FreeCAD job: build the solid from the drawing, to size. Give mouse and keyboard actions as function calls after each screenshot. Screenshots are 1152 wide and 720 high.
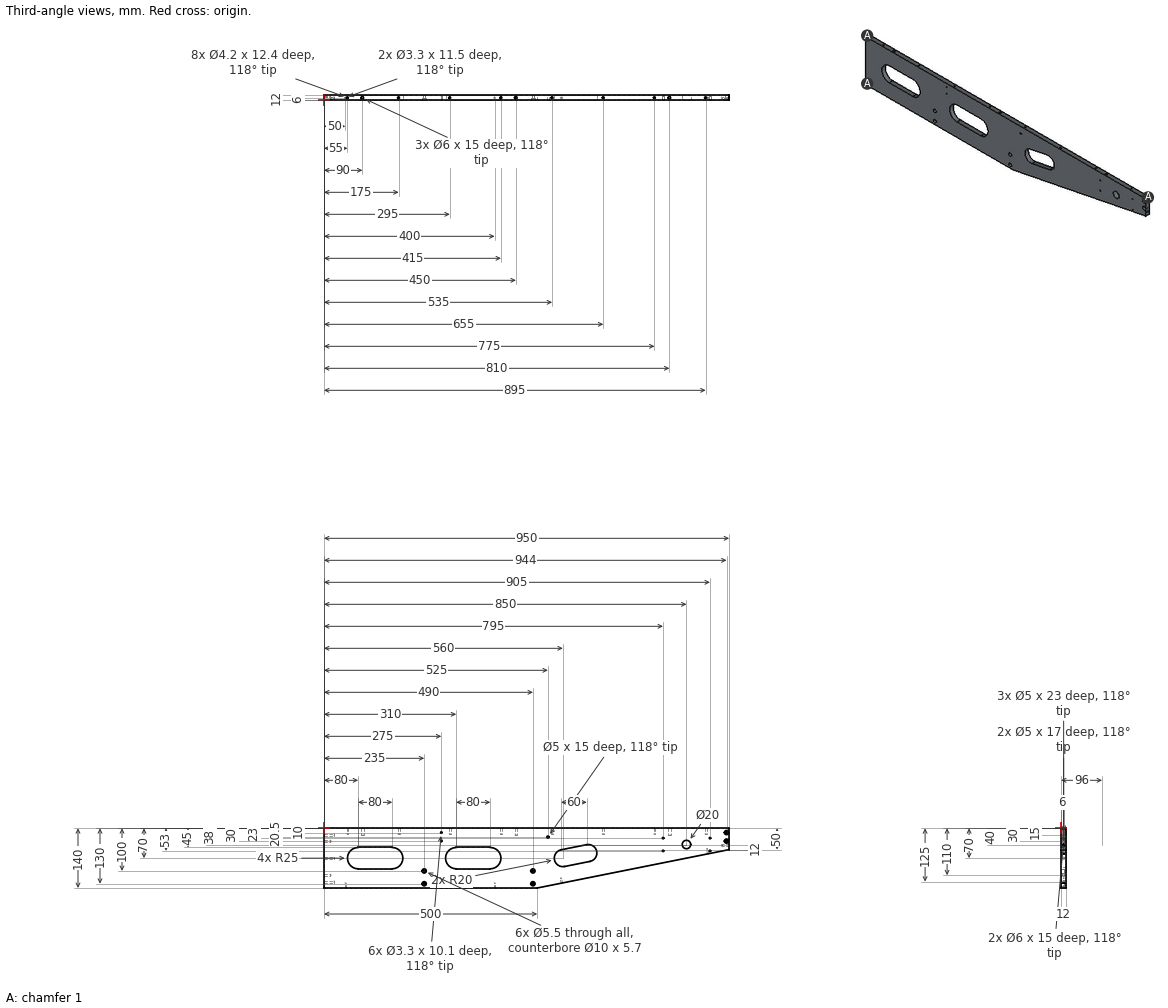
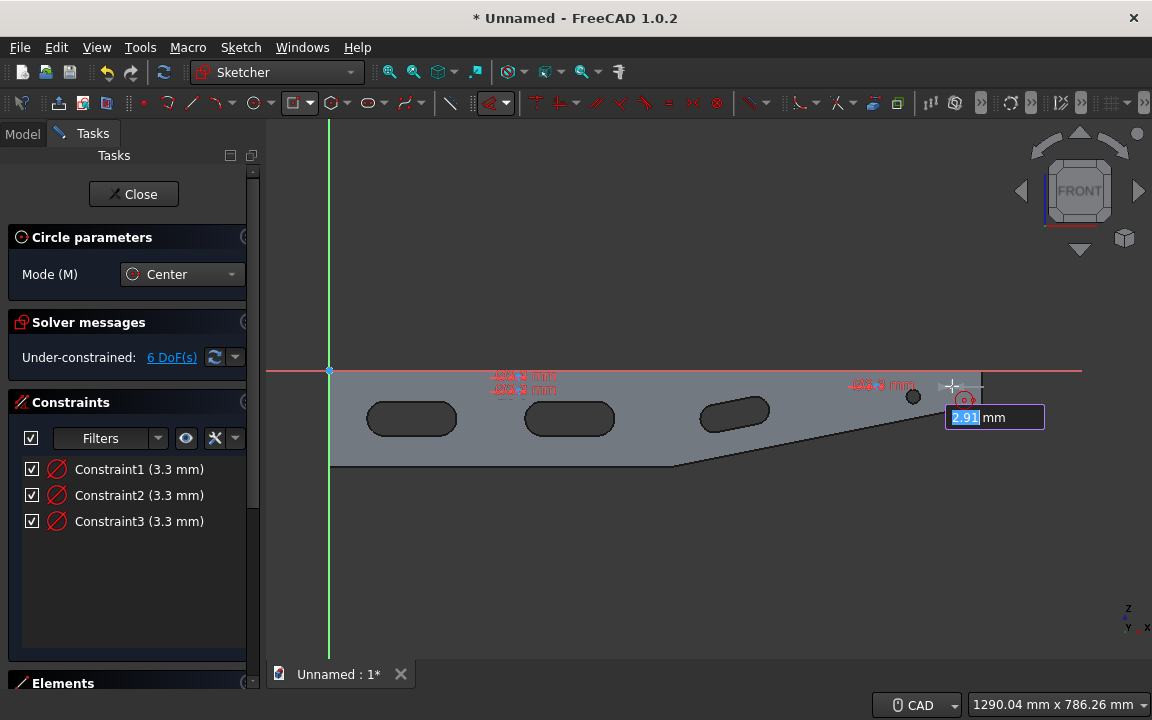
text(3.3)
key(Return)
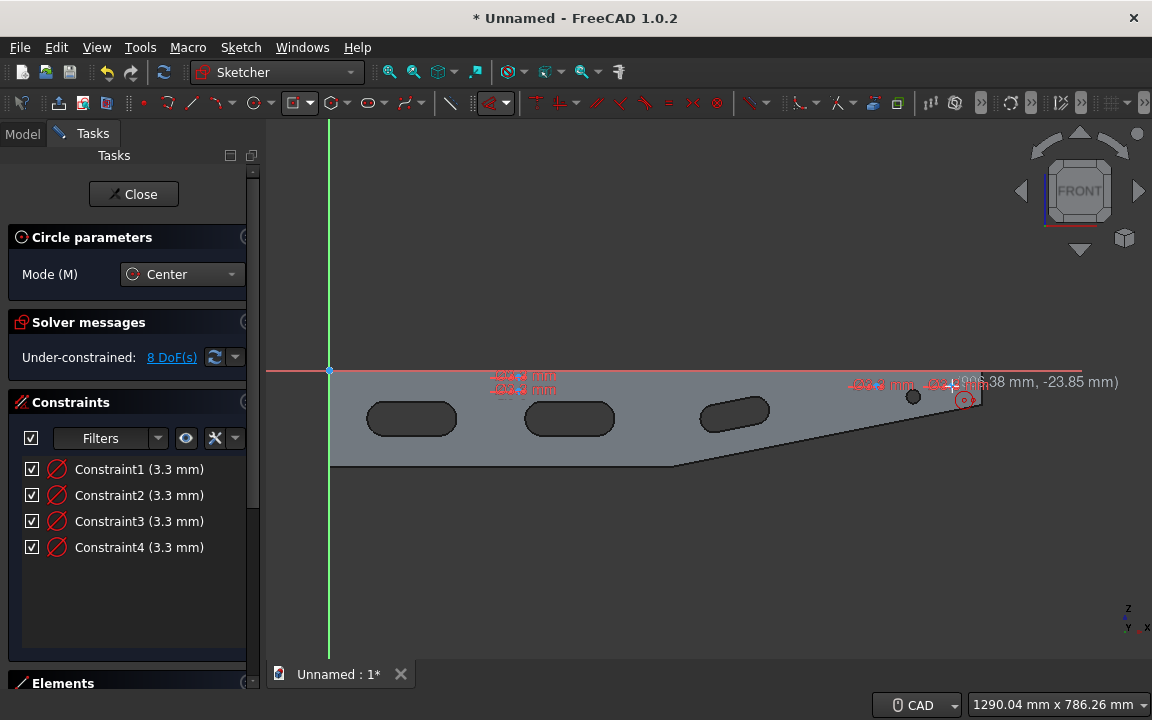
scroll(876, 407, up, 15)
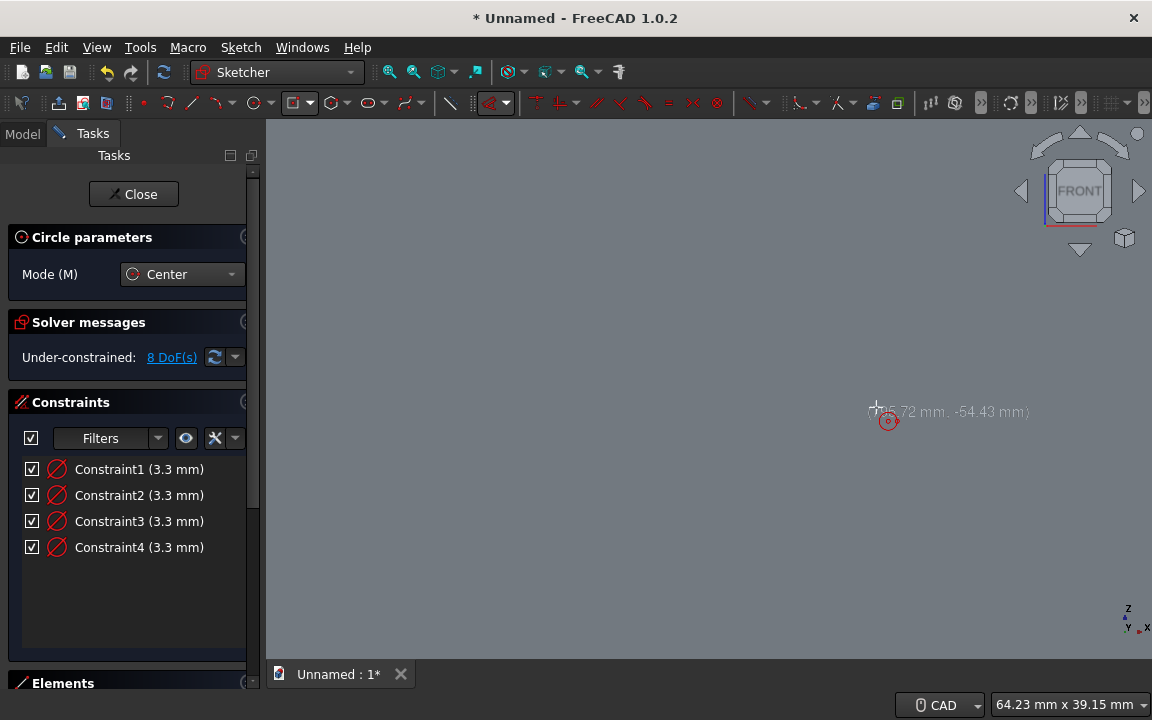
scroll(876, 407, down, 15)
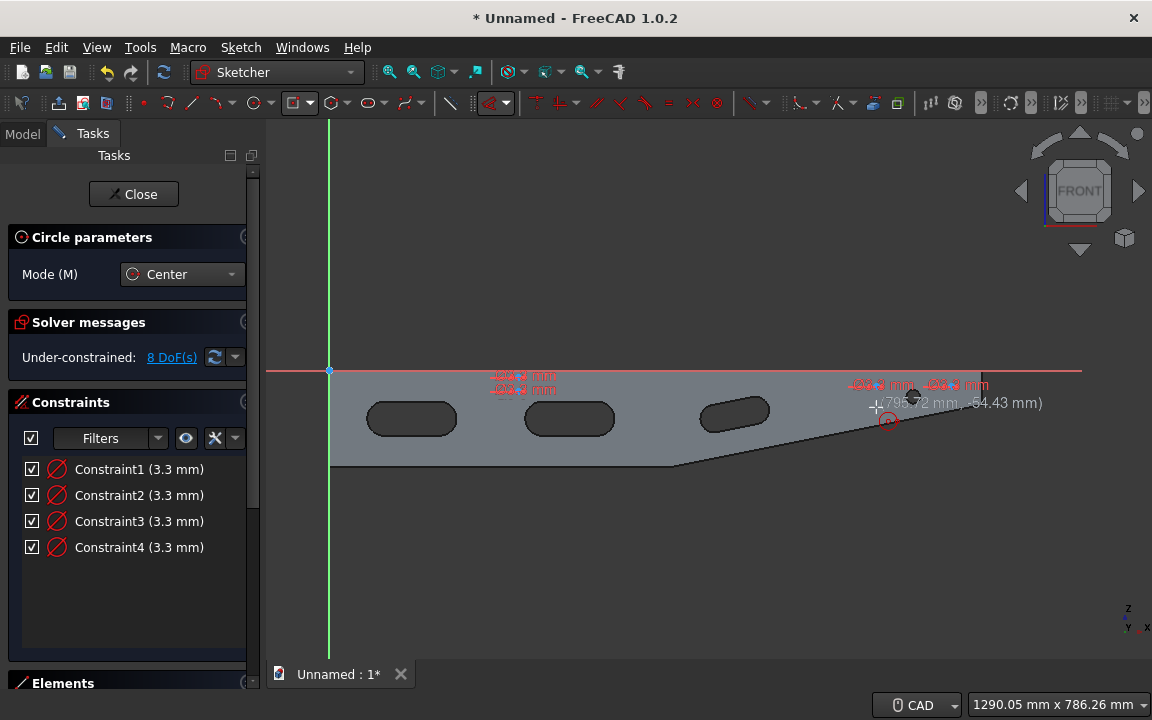
click(876, 407)
move(876, 406)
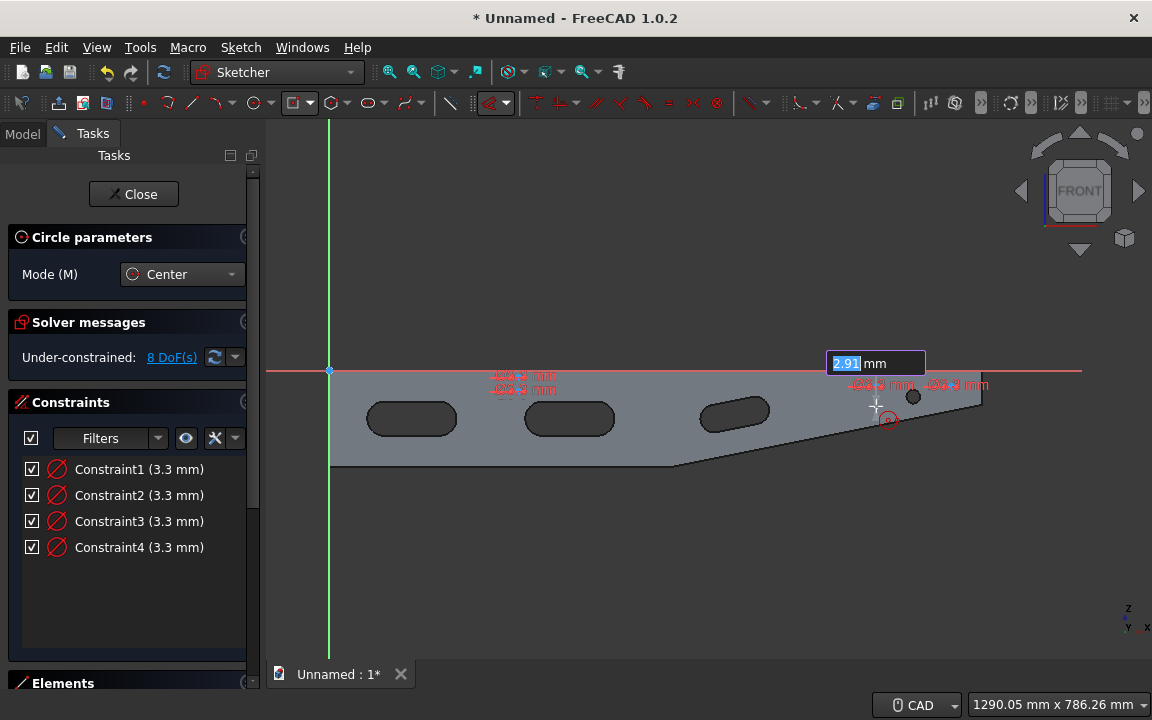
text(3.3)
key(Return)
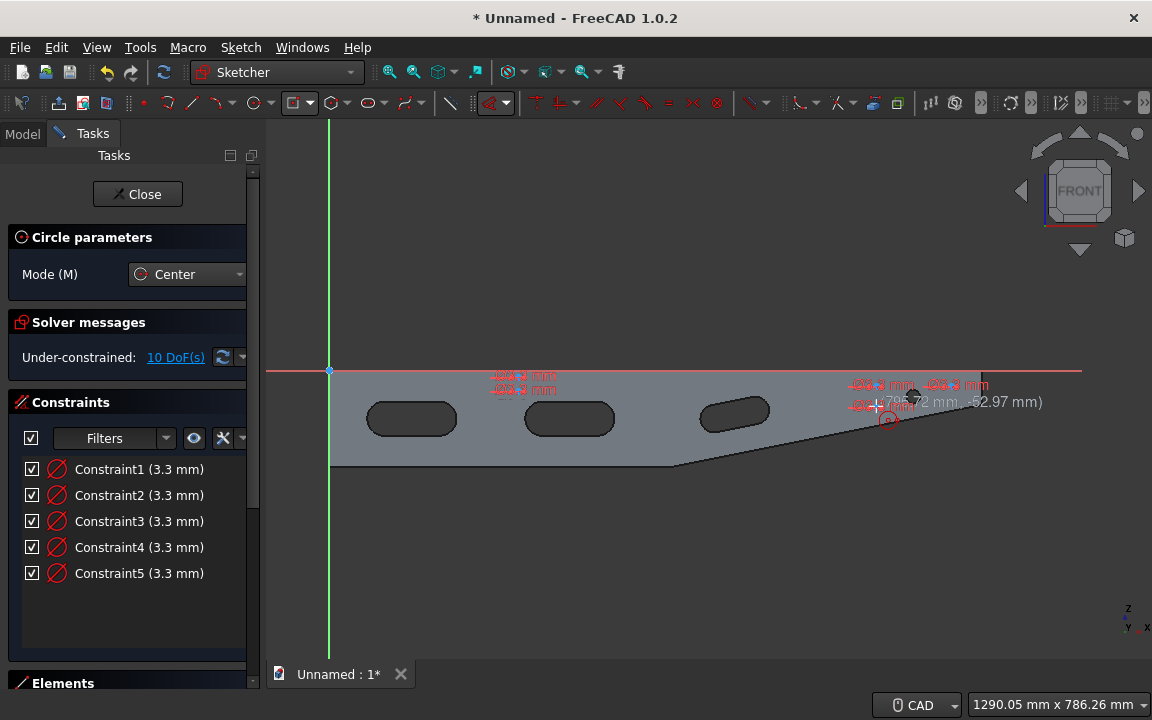
scroll(951, 407, up, 15)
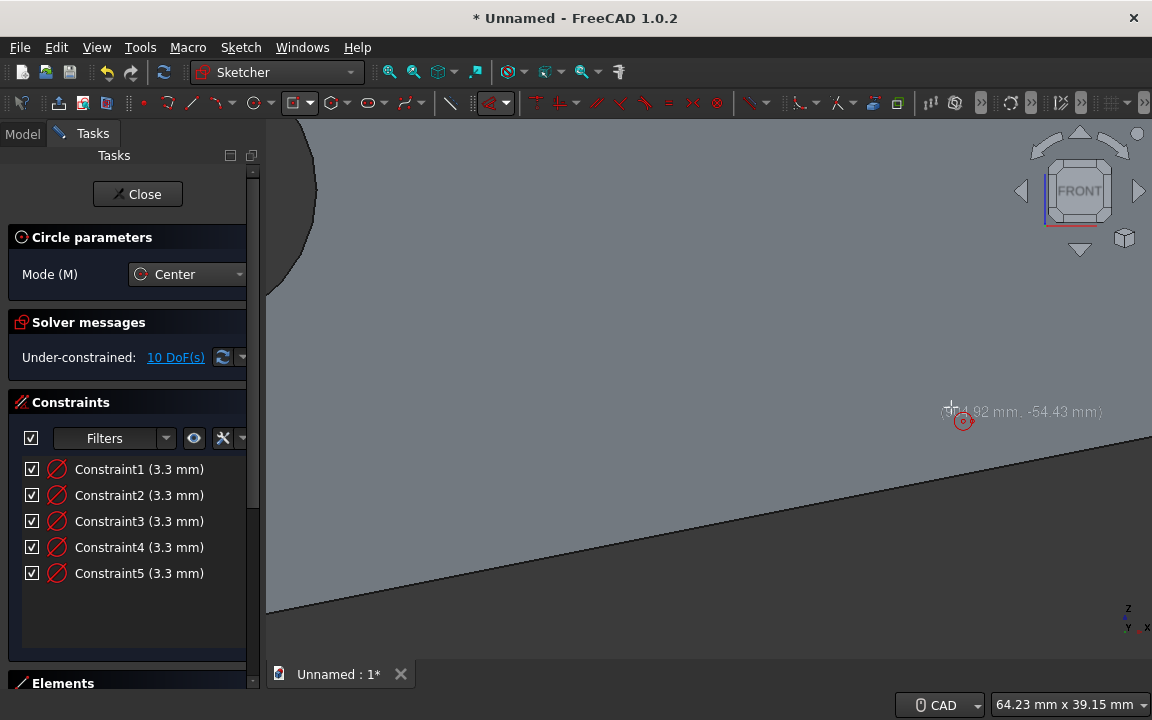
scroll(951, 407, down, 15)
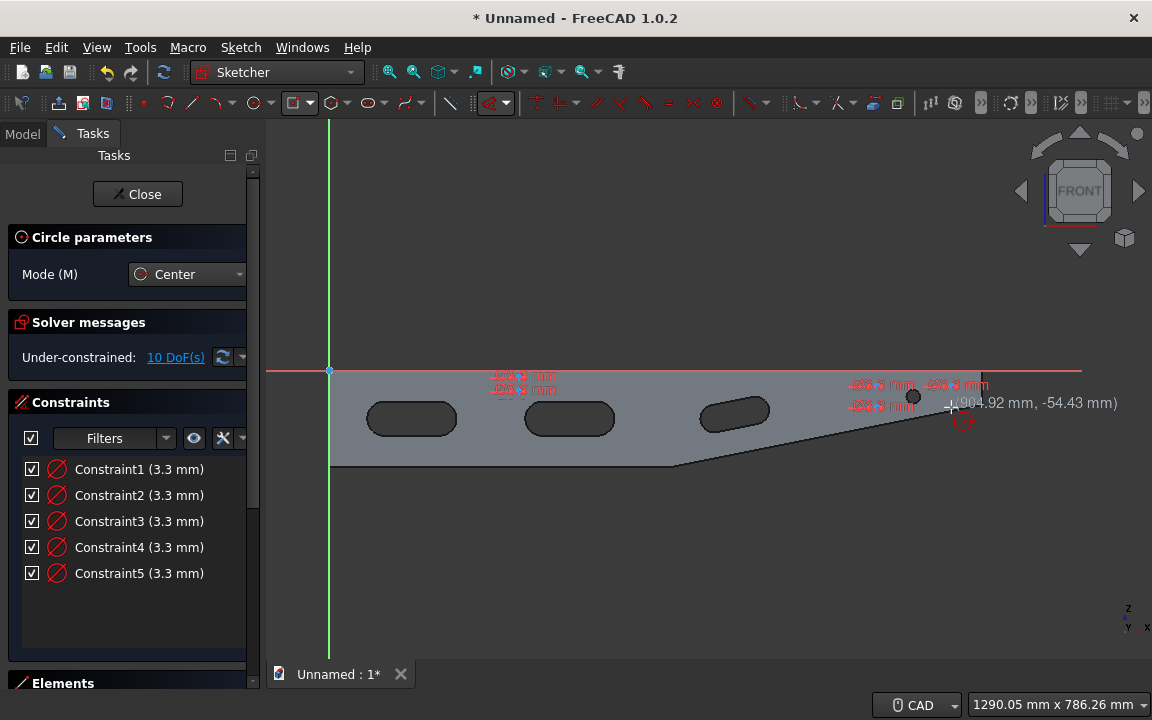
click(951, 407)
move(952, 406)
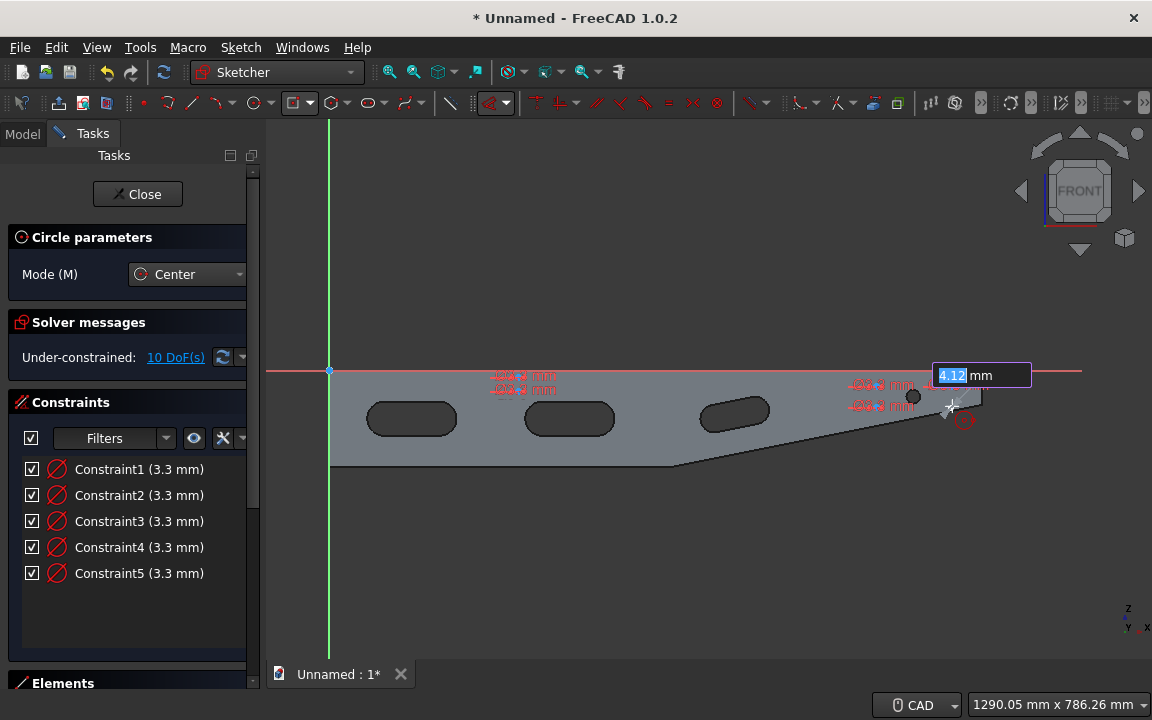
text(3.3)
key(Return)
key(Escape)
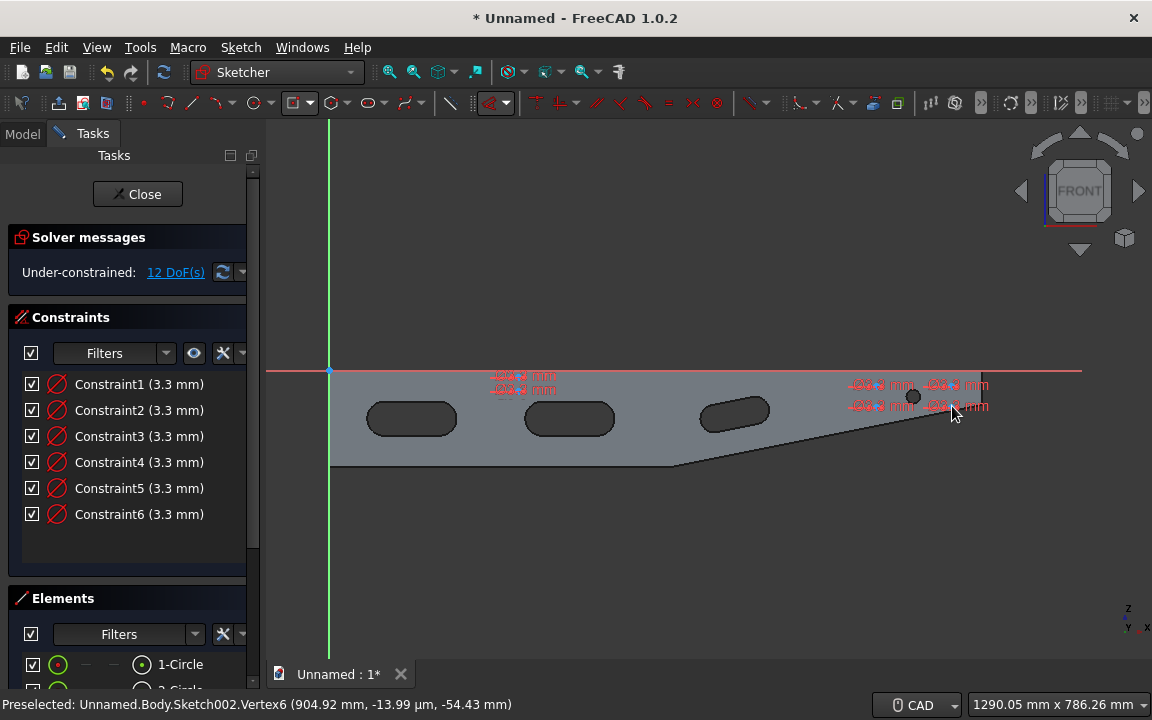
click(518, 378)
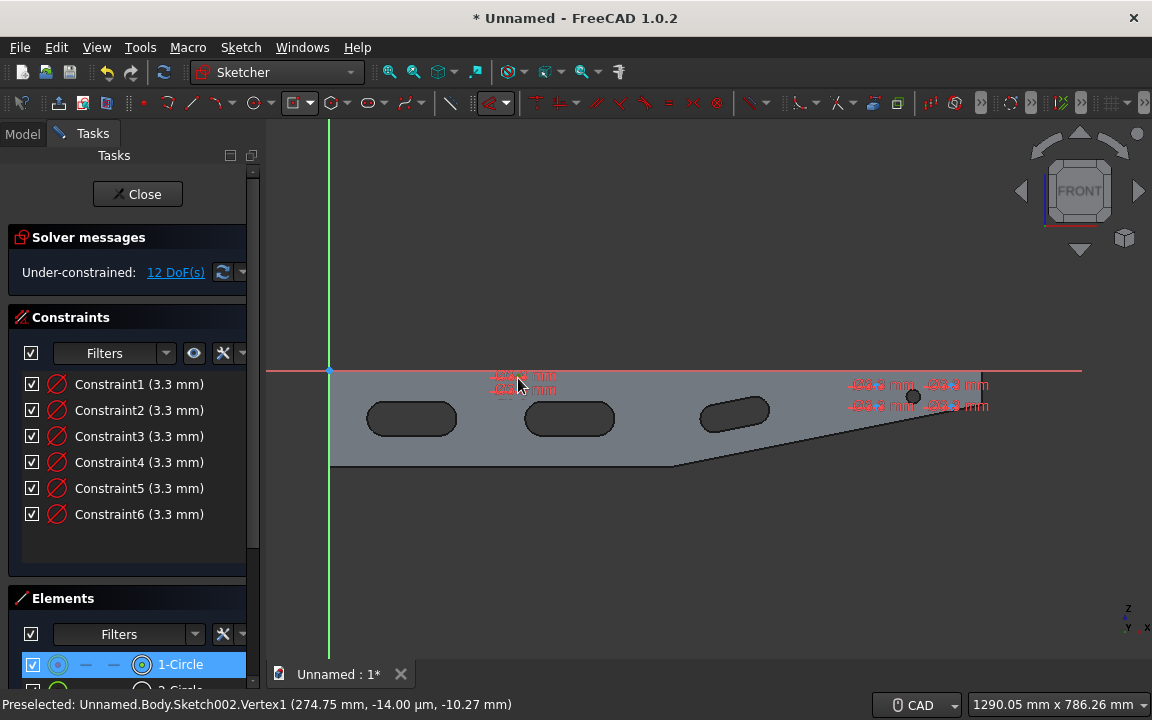
click(518, 392)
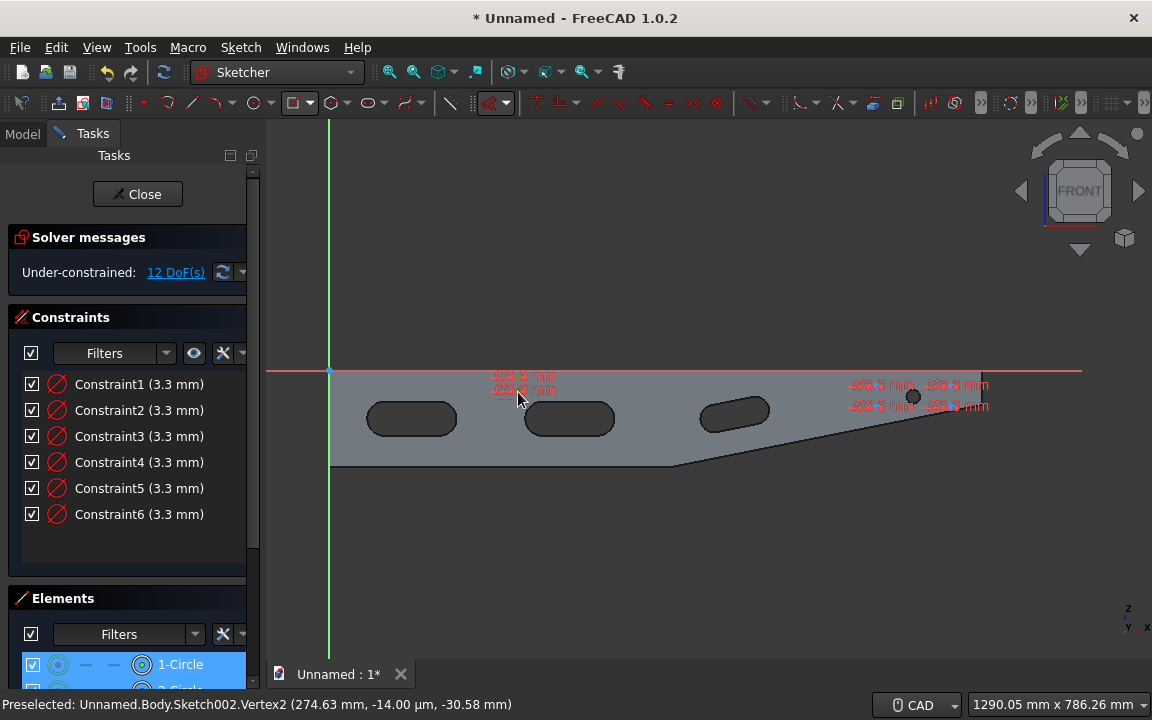
key(v)